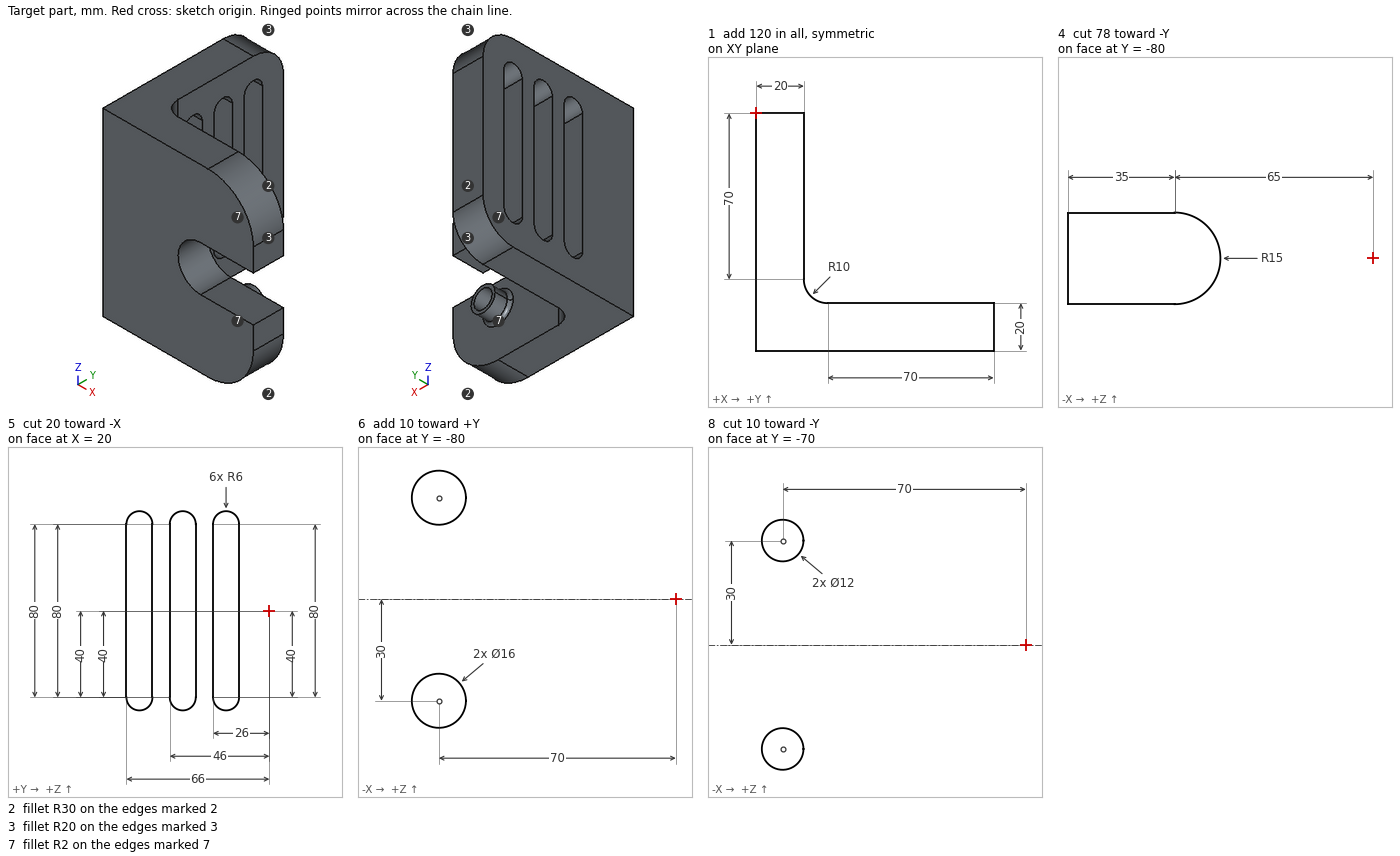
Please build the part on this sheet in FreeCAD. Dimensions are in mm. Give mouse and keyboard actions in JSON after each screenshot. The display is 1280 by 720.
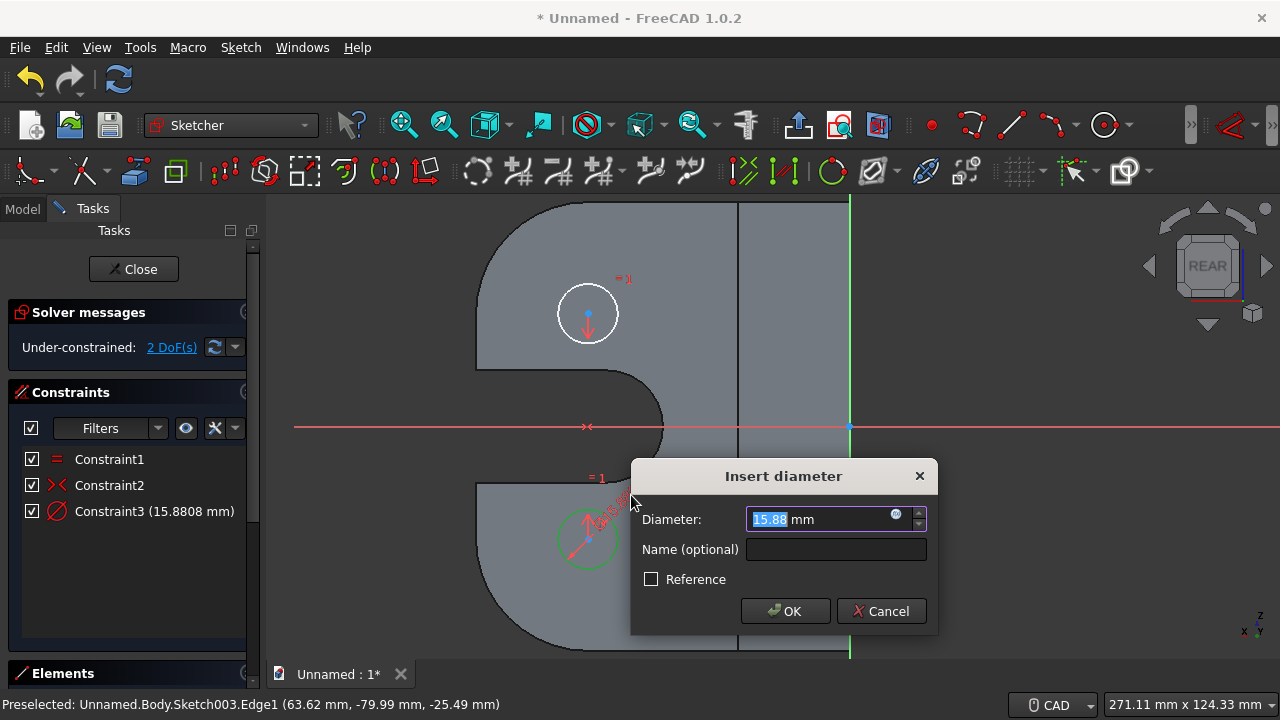
{"action": "type", "text": "16"}
{"action": "key", "text": "Return"}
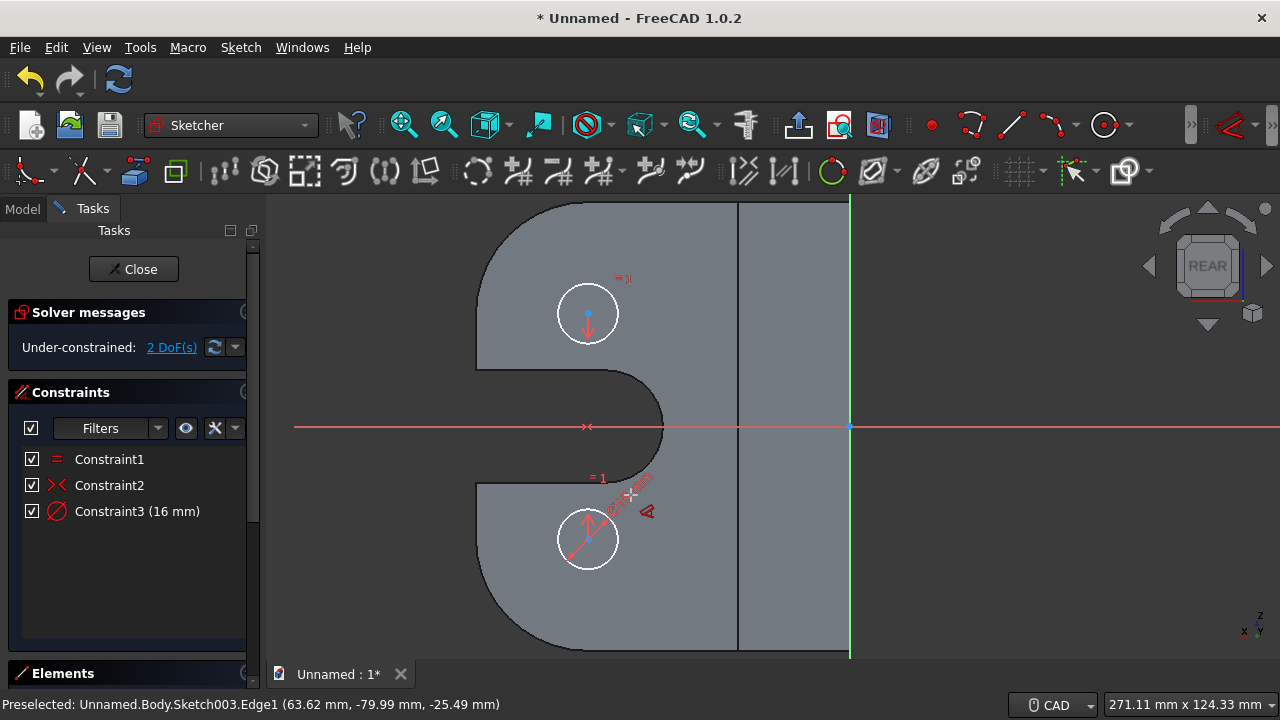
{"action": "left_click", "coordinate": [588, 539]}
{"action": "left_click", "coordinate": [719, 573]}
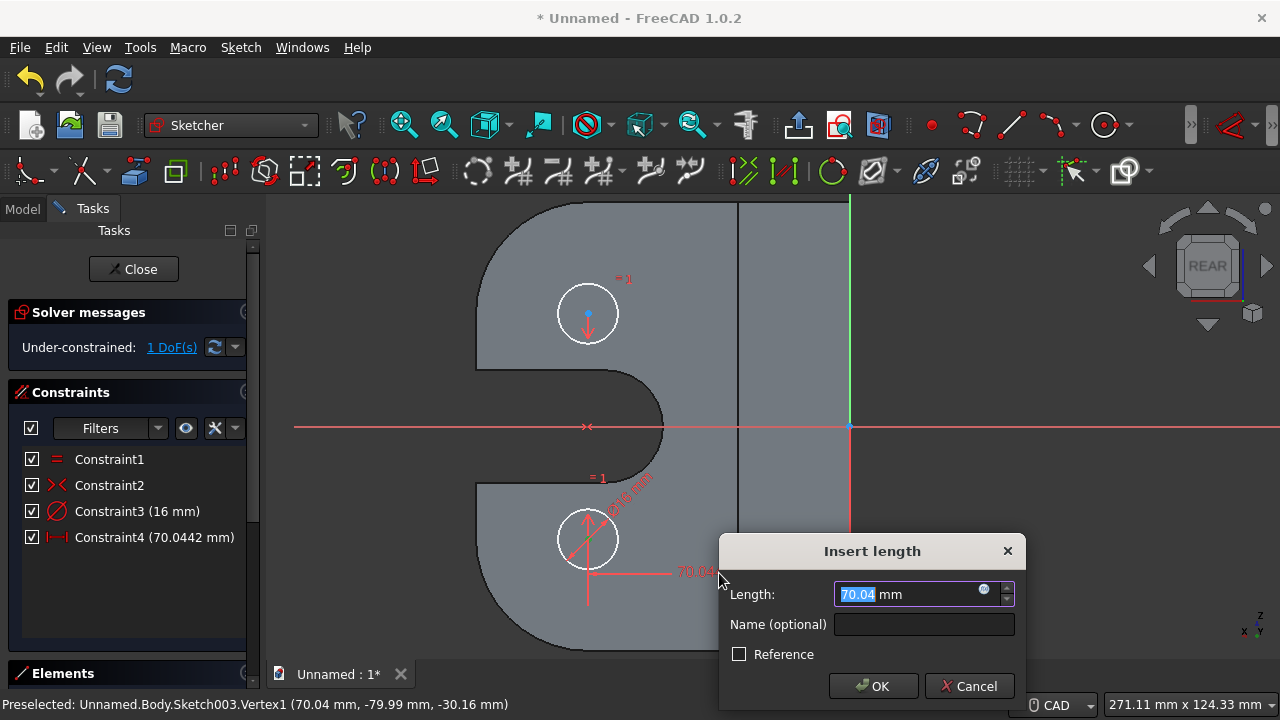
{"action": "type", "text": "70"}
{"action": "key", "text": "Return"}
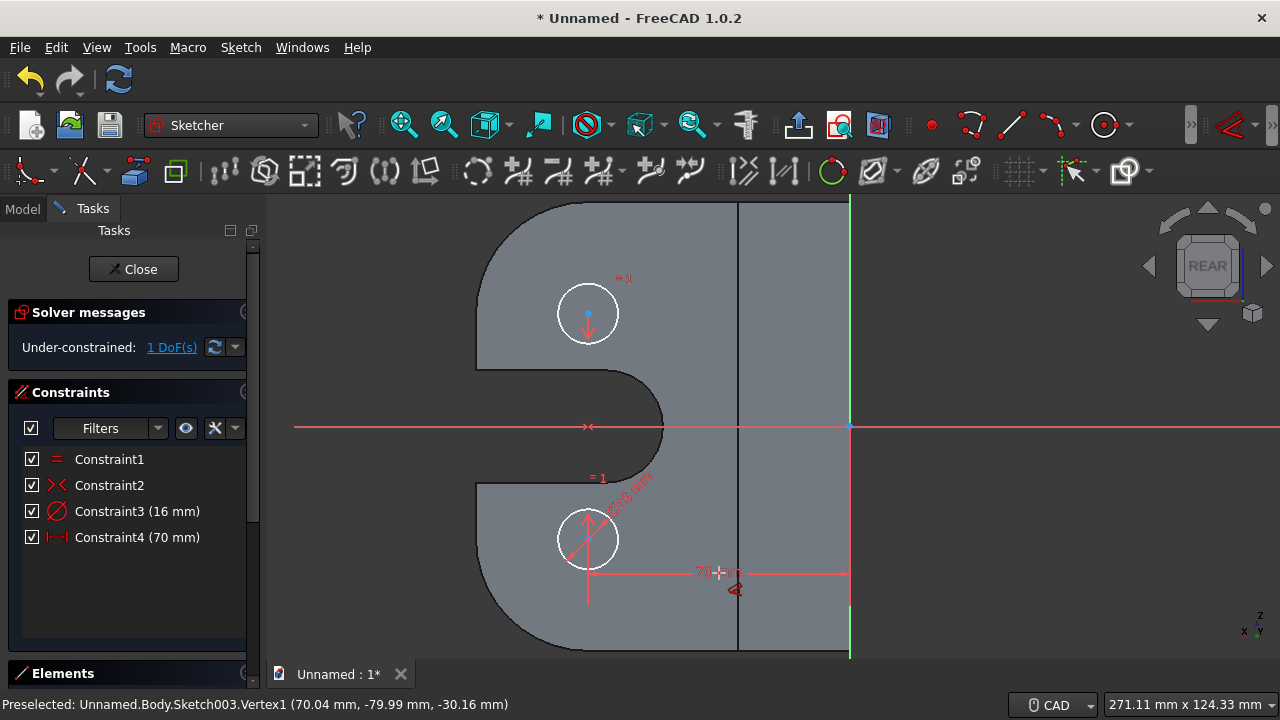
{"action": "left_click", "coordinate": [588, 539]}
{"action": "left_click", "coordinate": [884, 483]}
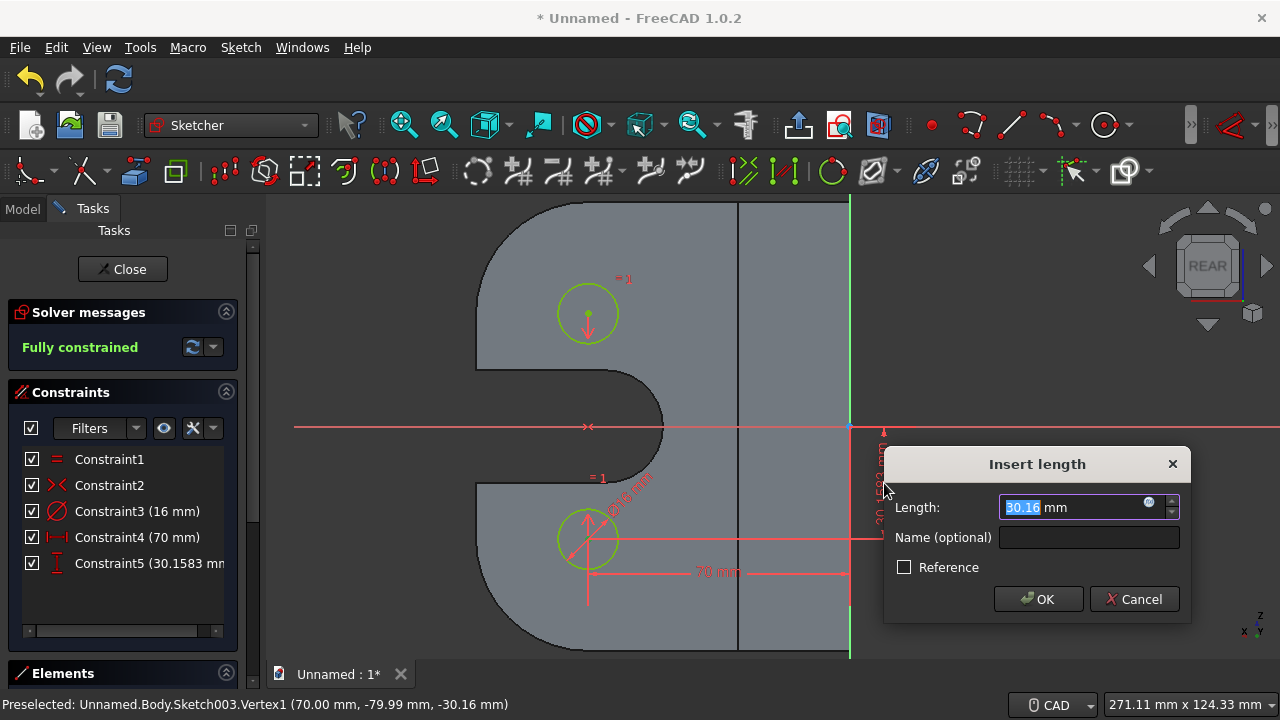
{"action": "type", "text": "30"}
{"action": "key", "text": "Return"}
{"action": "key", "text": "Escape"}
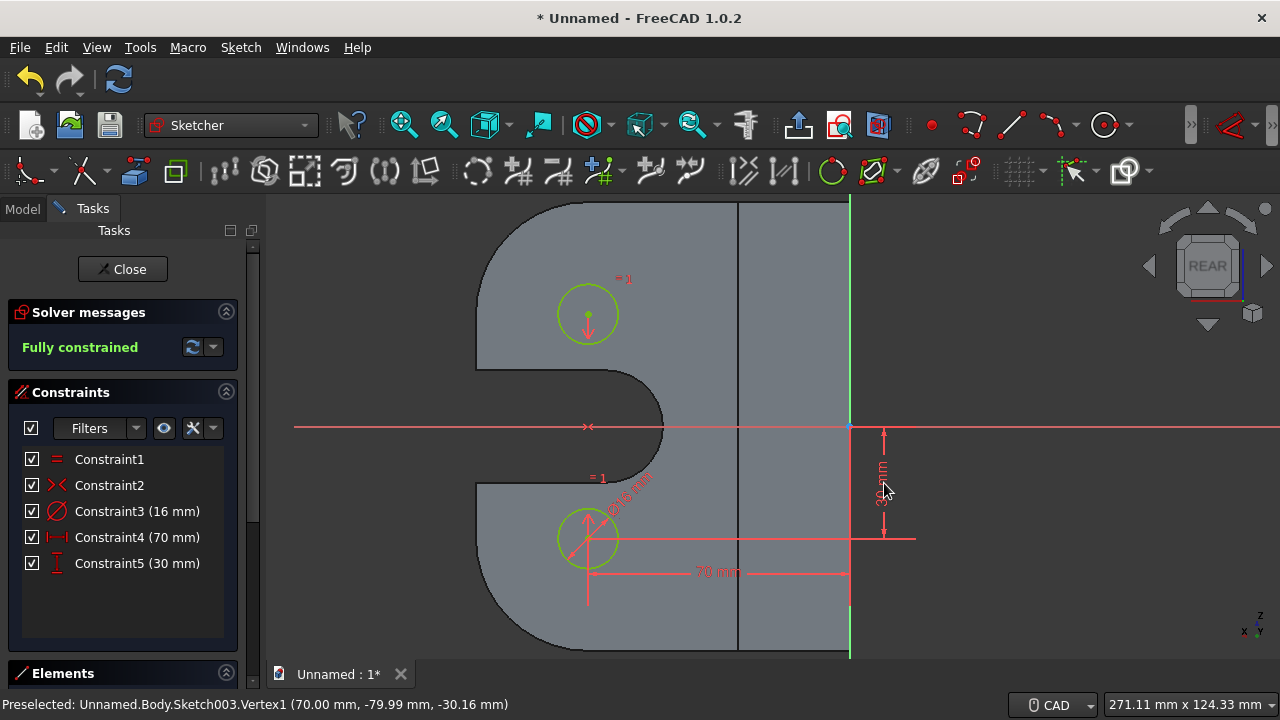
{"action": "left_click", "coordinate": [123, 269]}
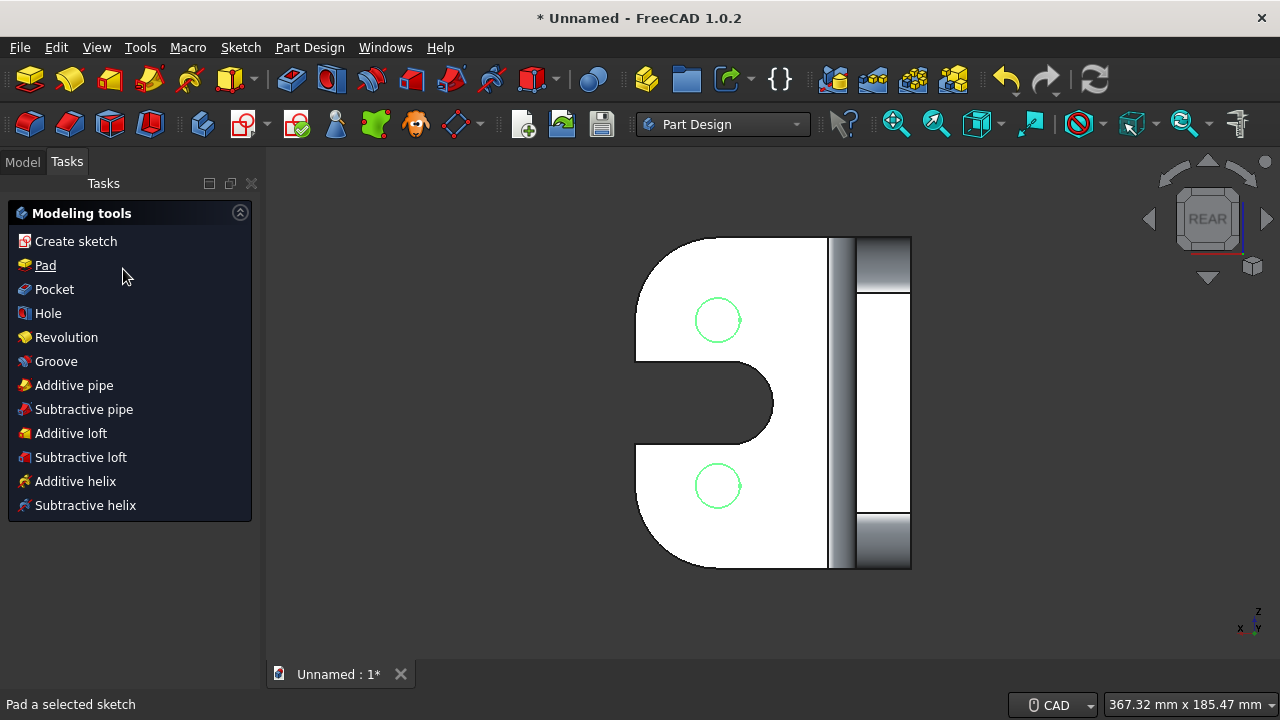
{"action": "left_click", "coordinate": [30, 80]}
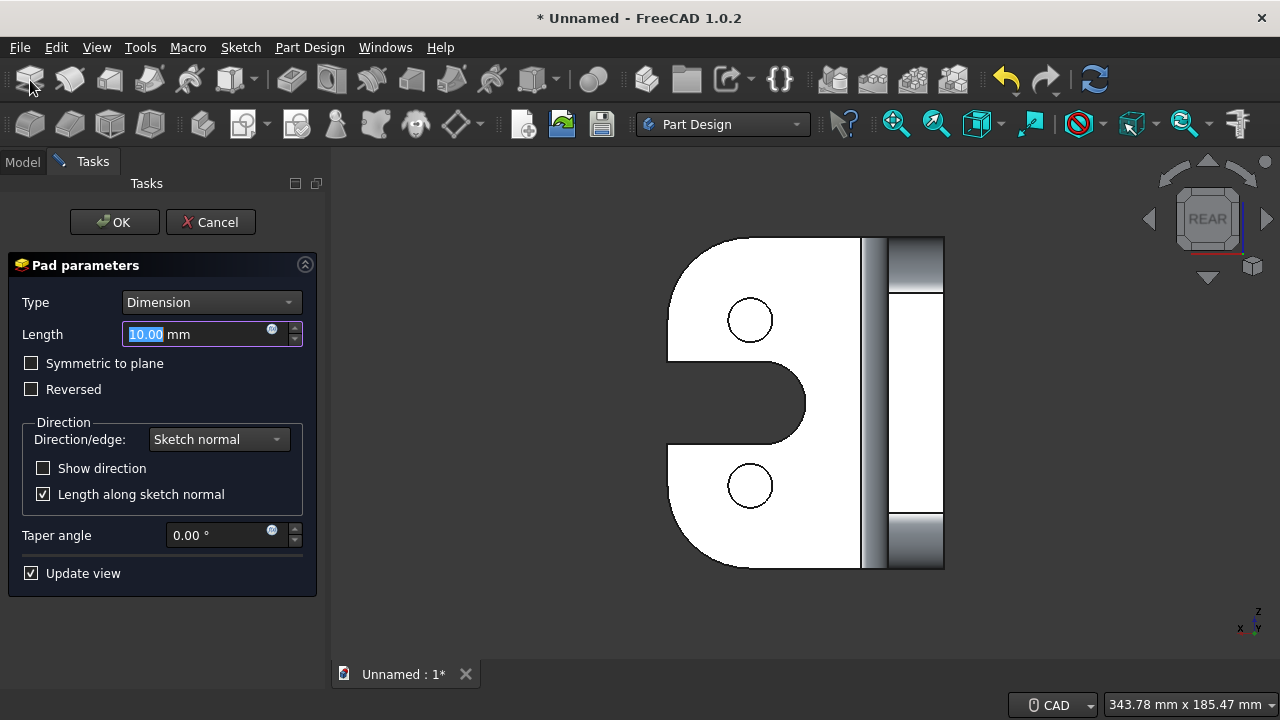
{"action": "type", "text": "10"}
{"action": "key", "text": "Tab"}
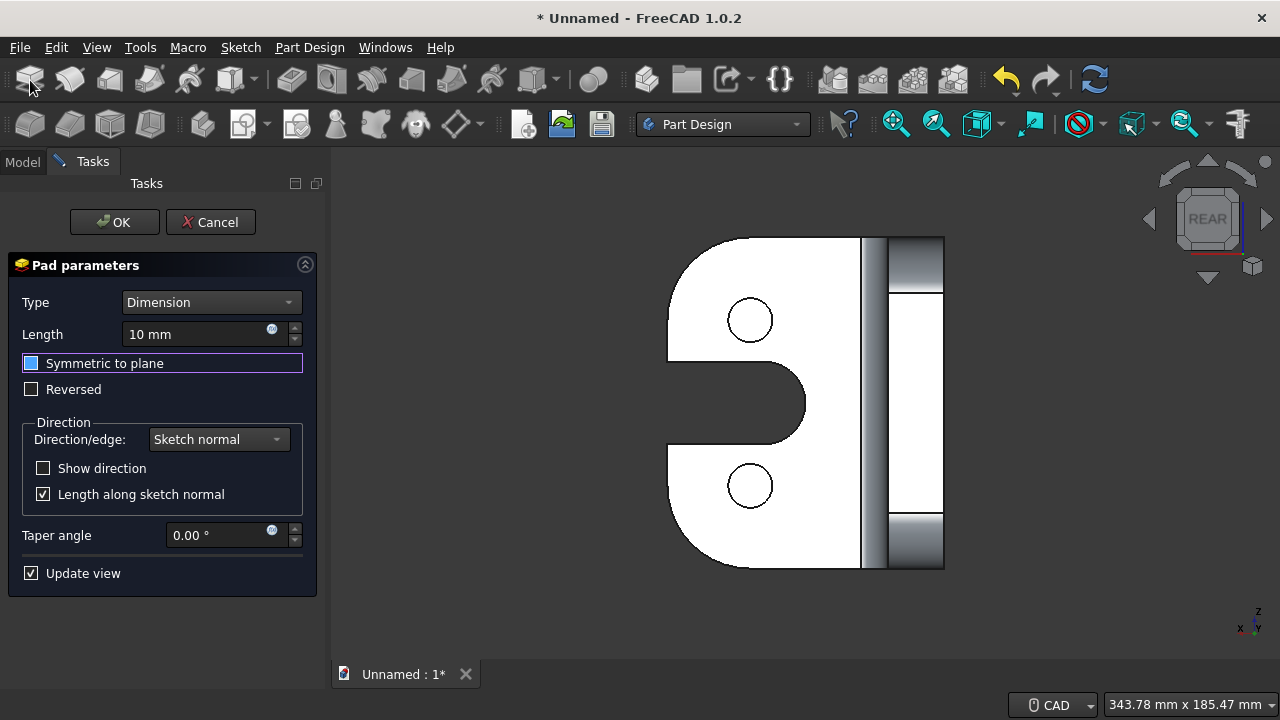
{"action": "left_click", "coordinate": [115, 222]}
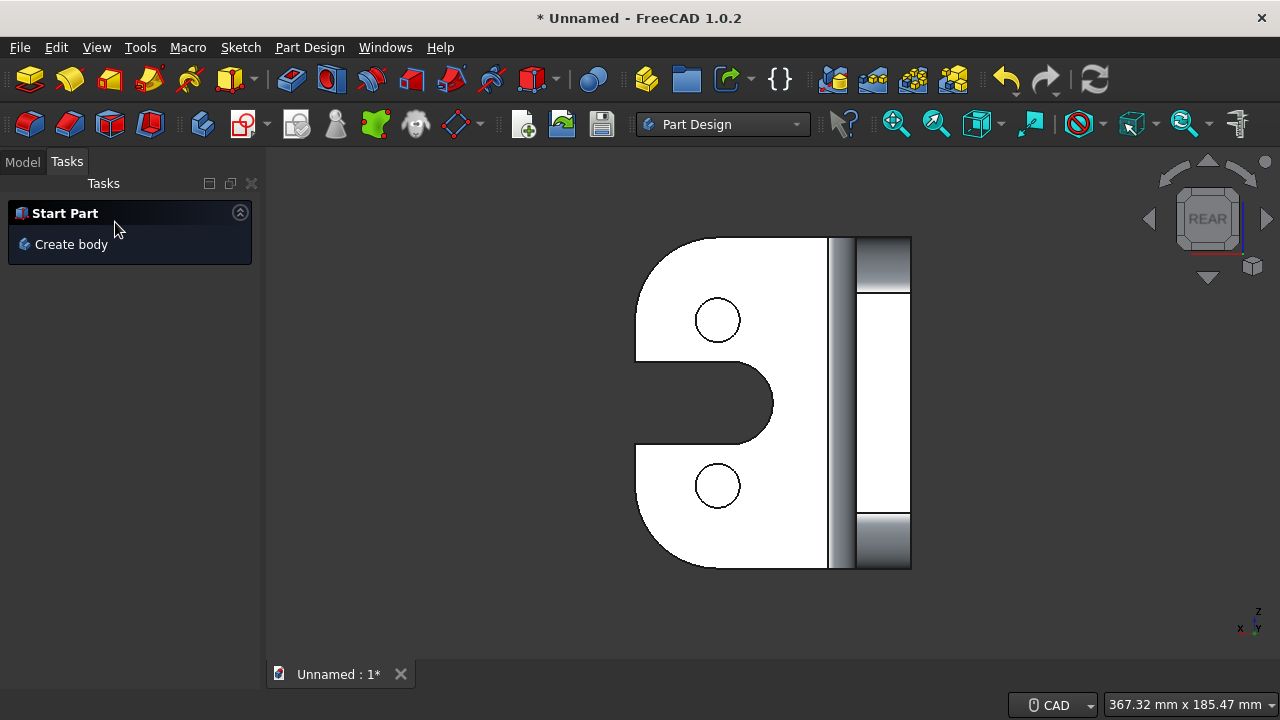
{"action": "key", "text": "0"}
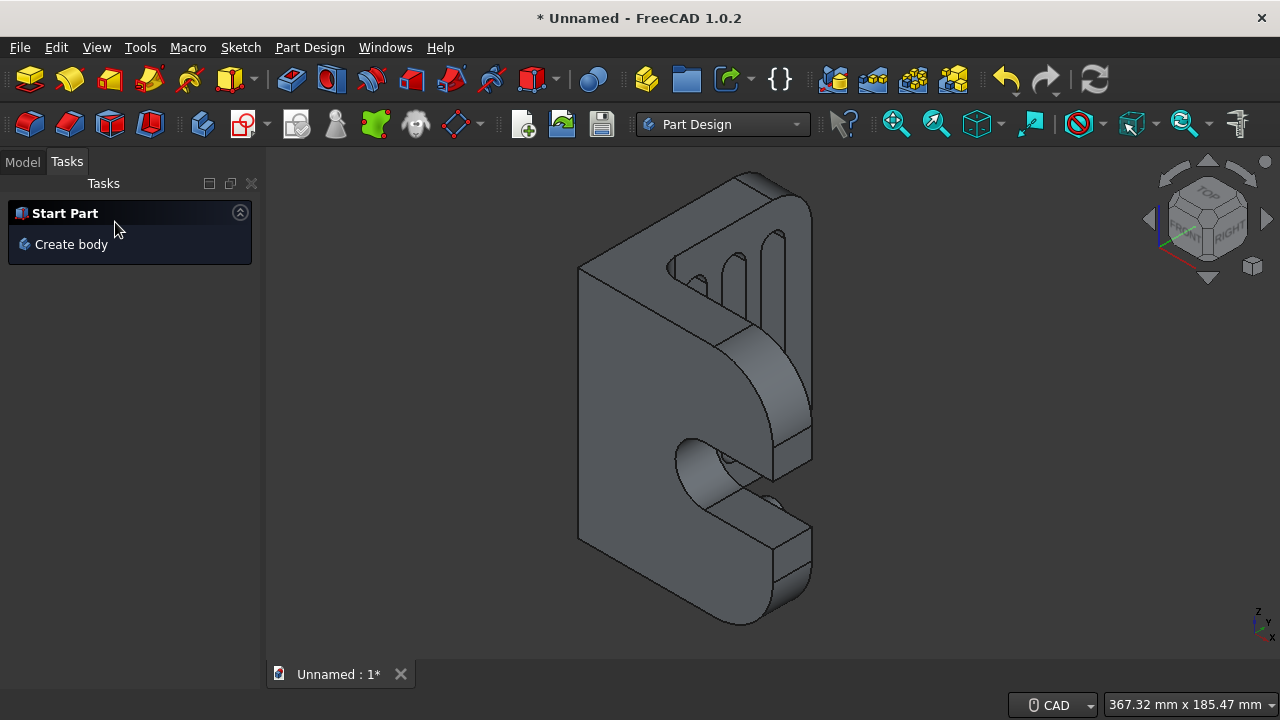
{"action": "key", "text": "2"}